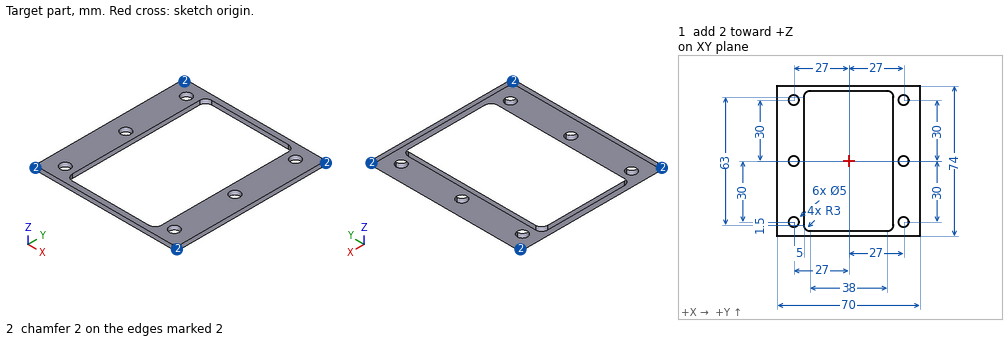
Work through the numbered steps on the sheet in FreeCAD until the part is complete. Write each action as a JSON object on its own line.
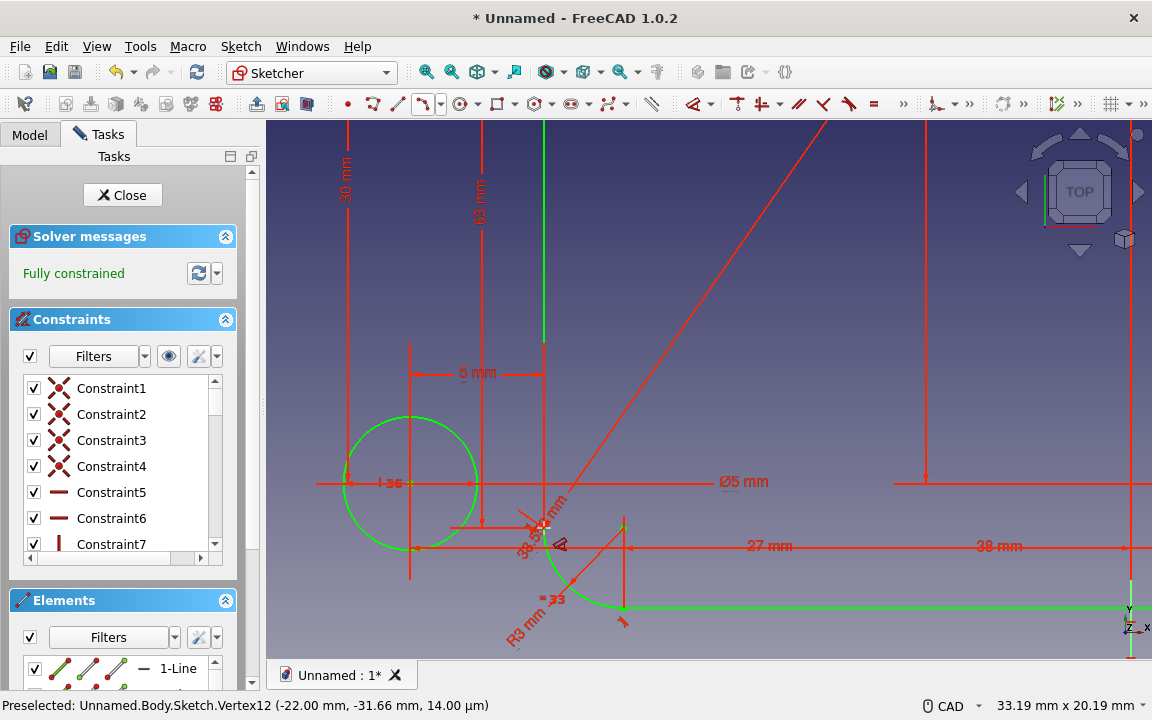
{"action": "left_click", "coordinate": [410, 484]}
{"action": "left_click", "coordinate": [376, 506]}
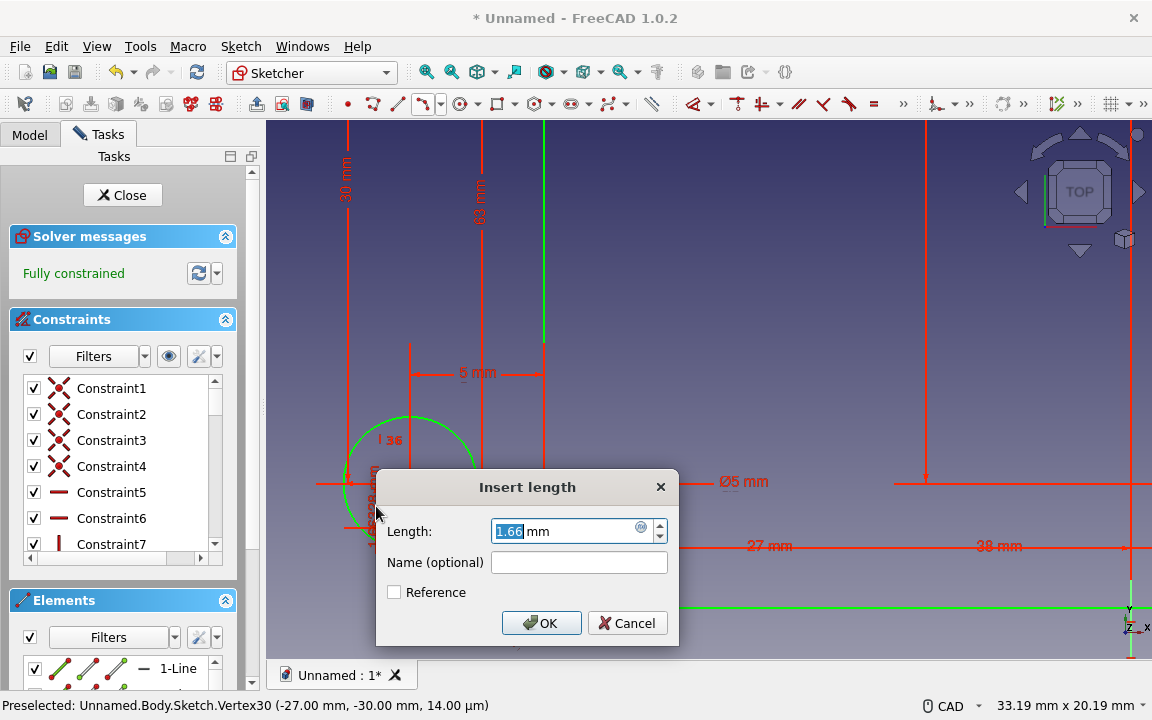
{"action": "type", "text": "1.5"}
{"action": "key", "text": "Return"}
{"action": "key", "text": "Escape"}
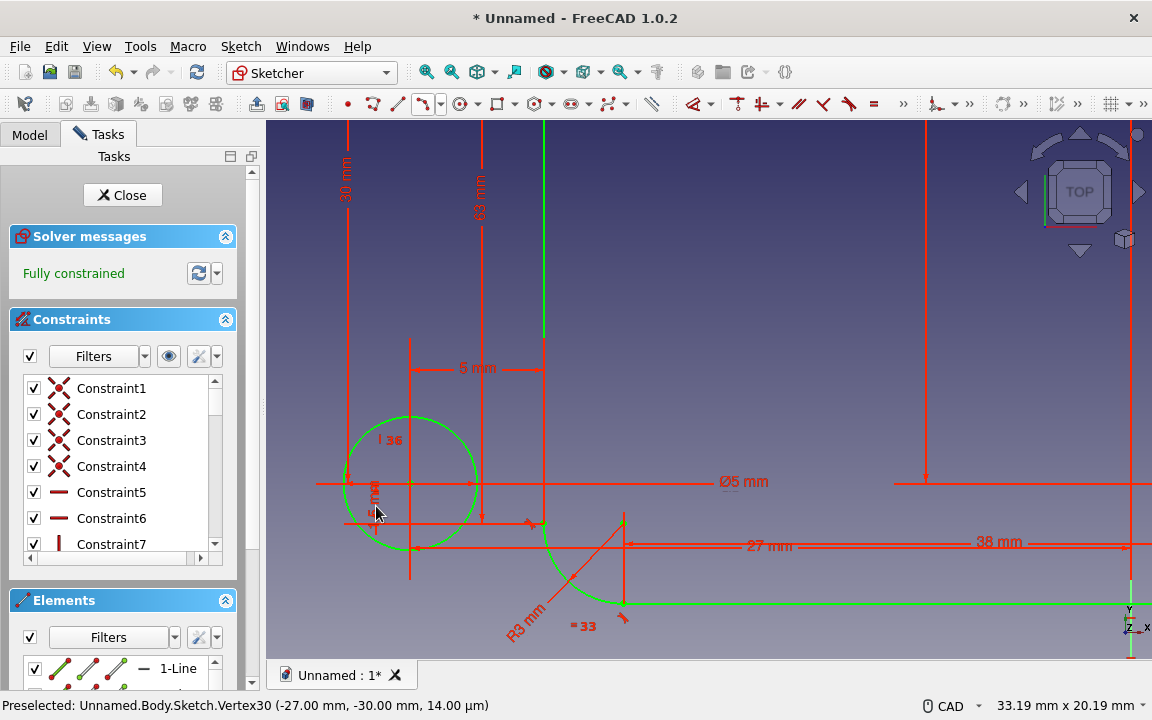
{"action": "left_click", "coordinate": [123, 195]}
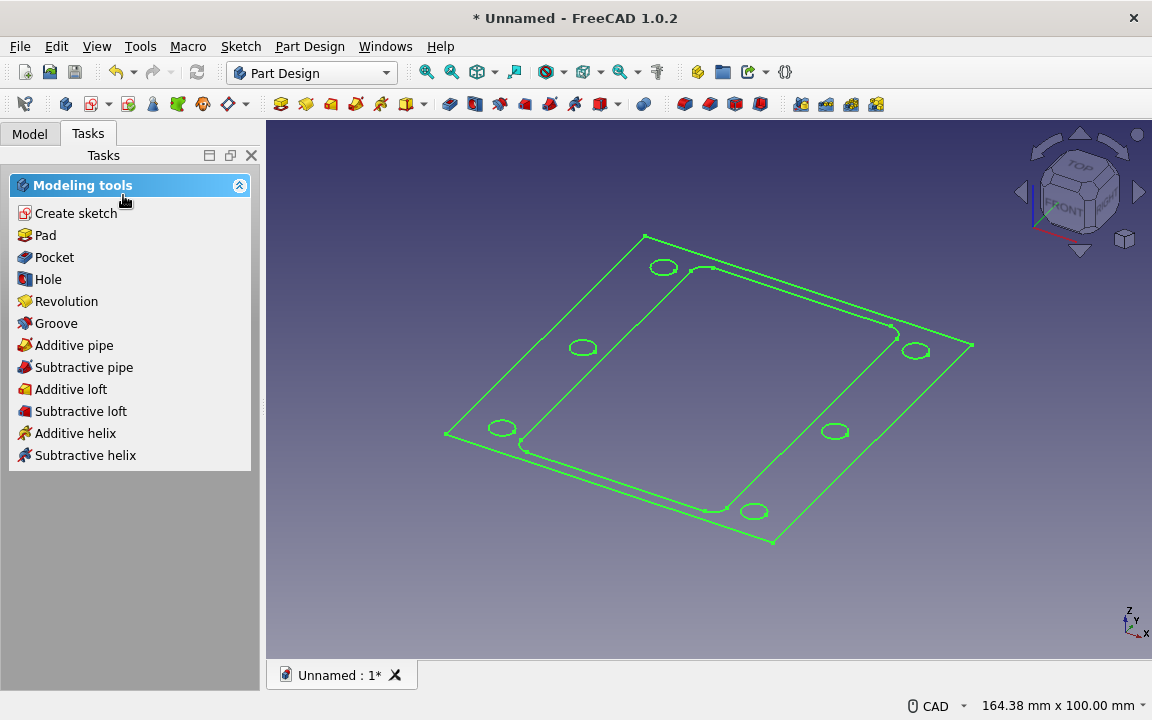
{"action": "left_click", "coordinate": [281, 104]}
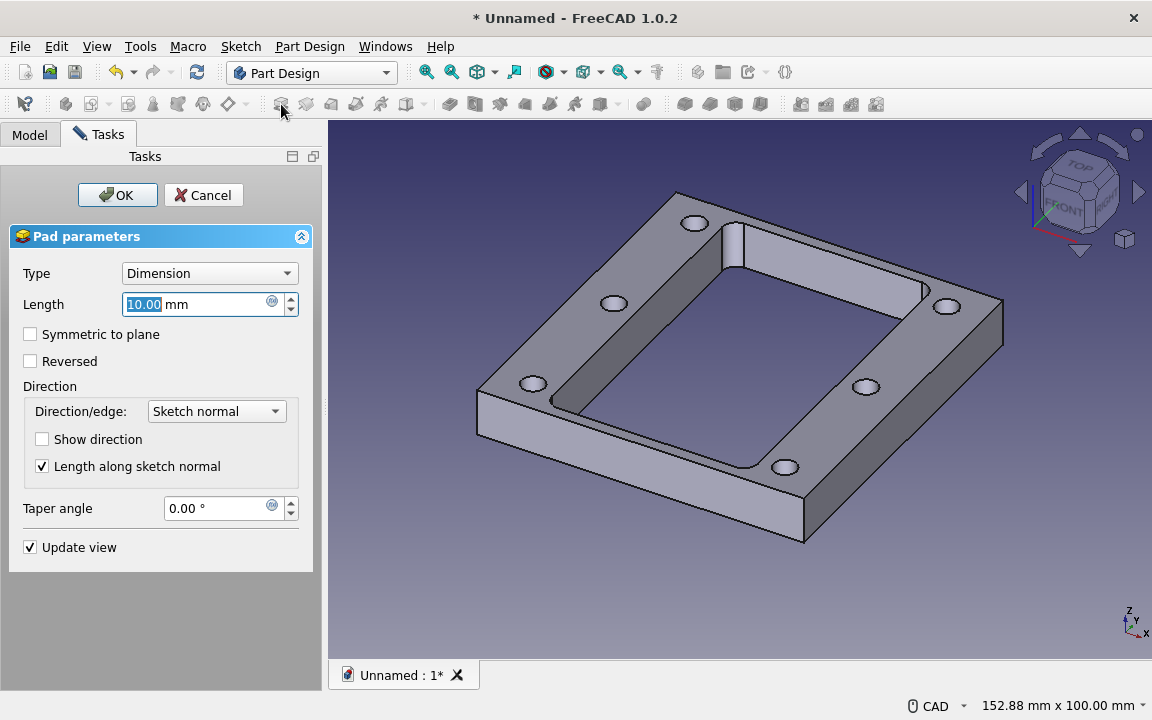
{"action": "type", "text": "2"}
{"action": "key", "text": "Tab"}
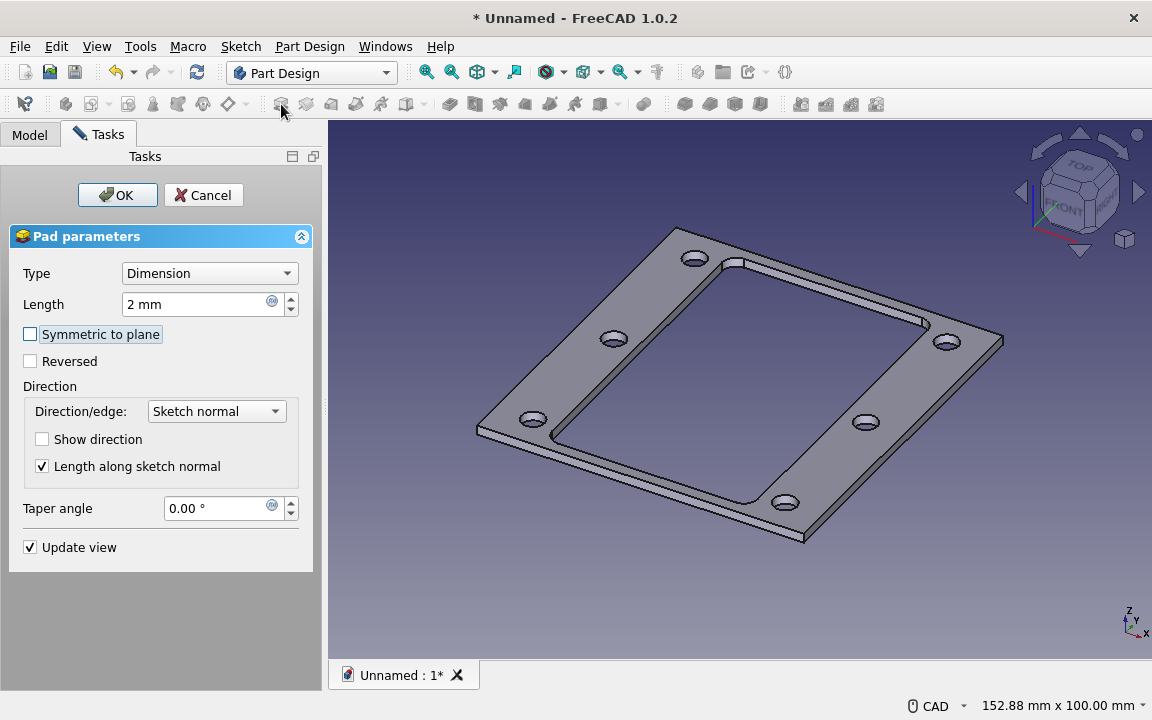
{"action": "left_click", "coordinate": [118, 195]}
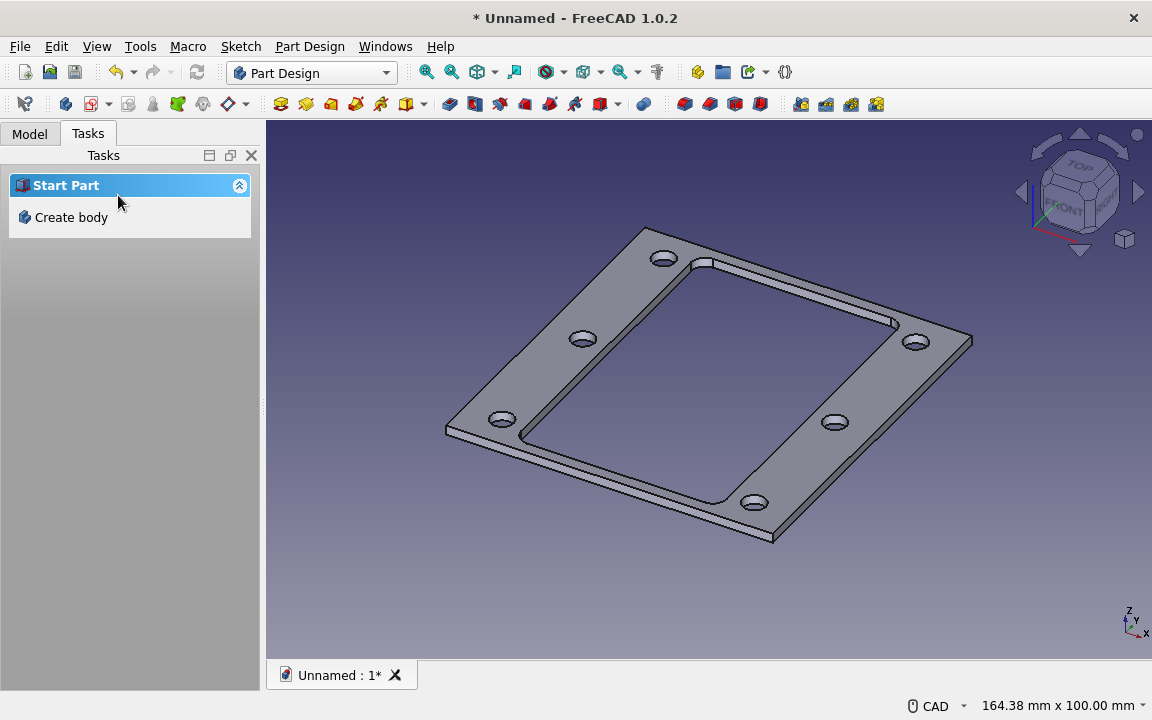
{"action": "left_click", "coordinate": [773, 539]}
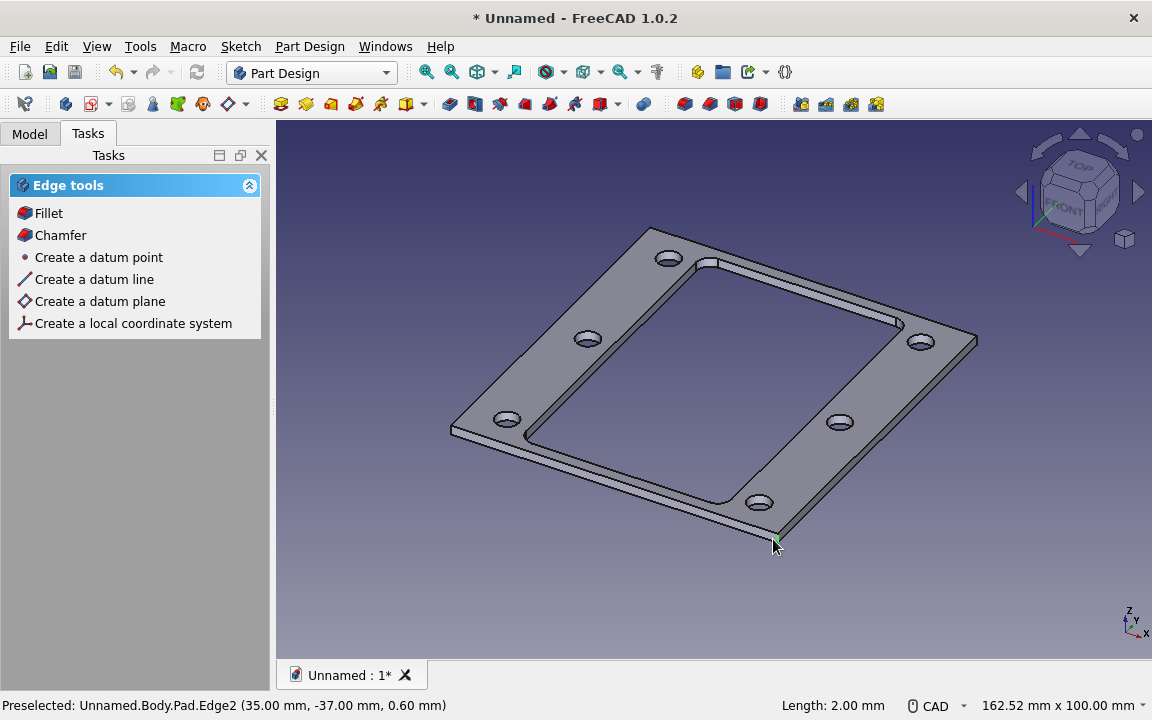
{"action": "scroll", "coordinate": [451, 429], "scroll_direction": "up", "scroll_amount": 7}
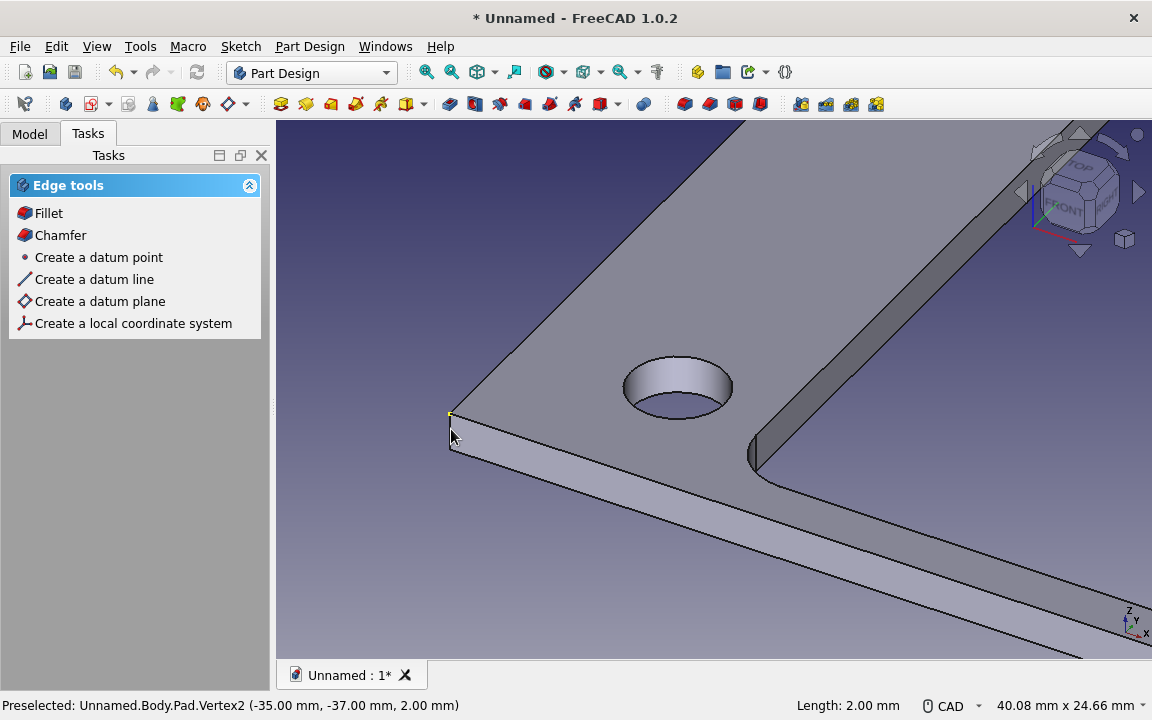
{"action": "left_click", "coordinate": [427, 72]}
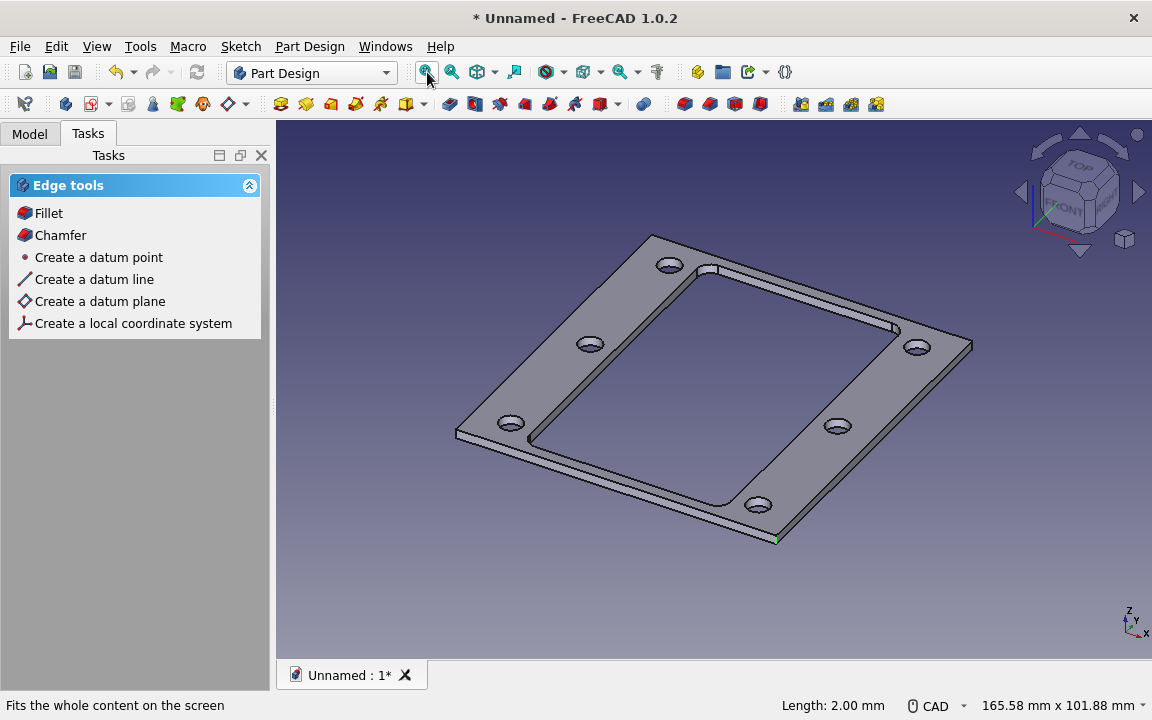
{"action": "key", "text": "0"}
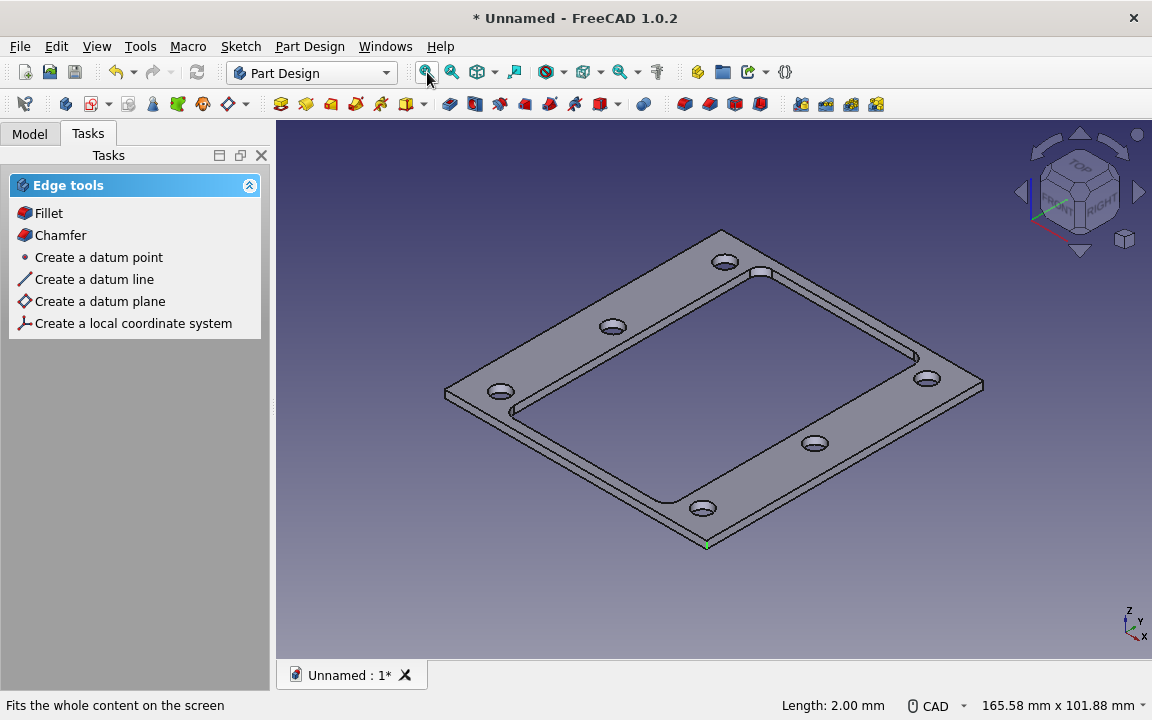
{"action": "scroll", "coordinate": [445, 393], "scroll_direction": "up", "scroll_amount": 7}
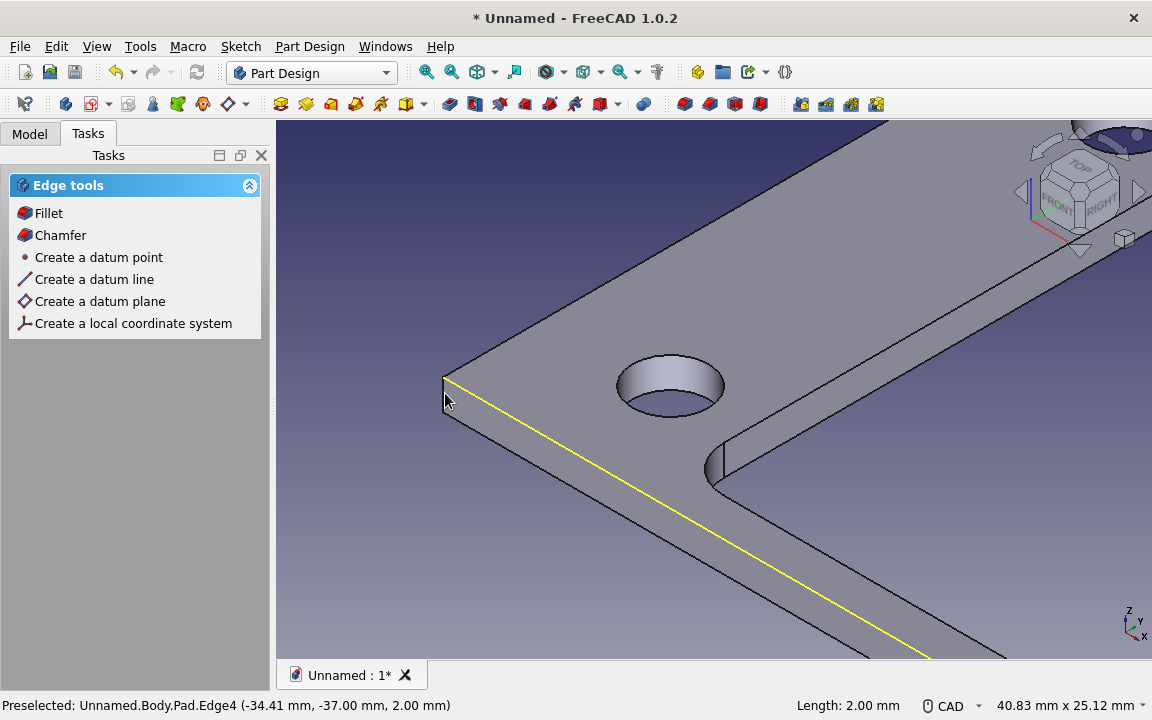
{"action": "left_click", "coordinate": [427, 72]}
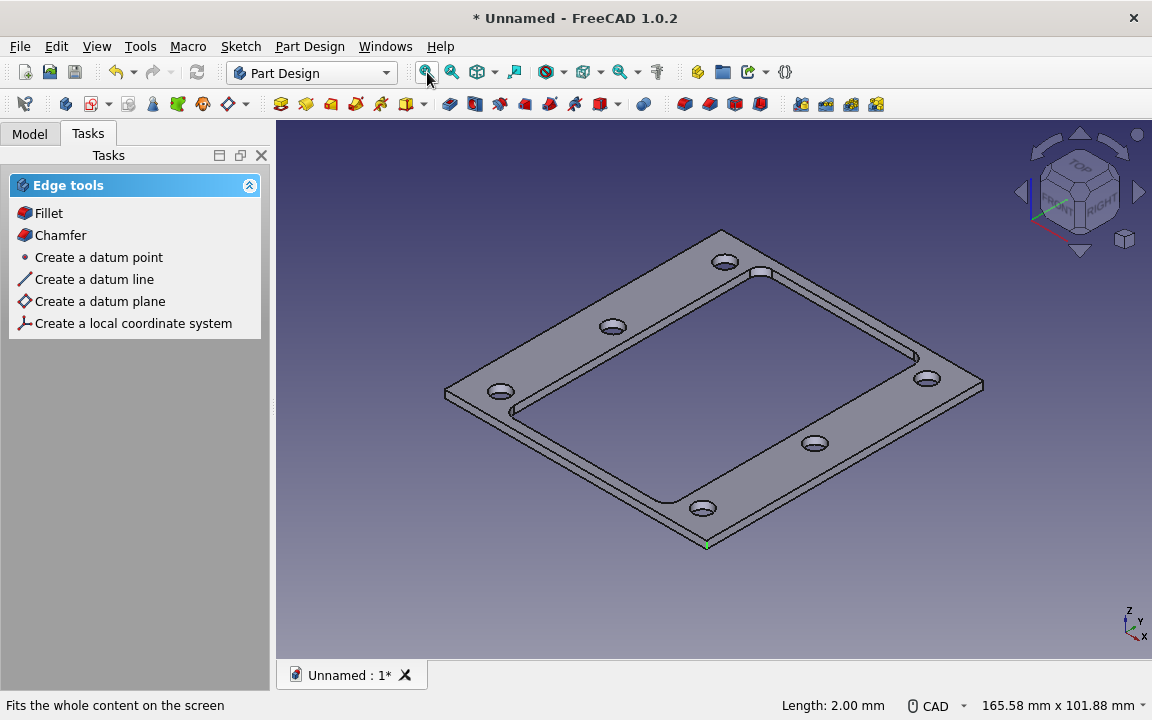
{"action": "key", "text": "2"}